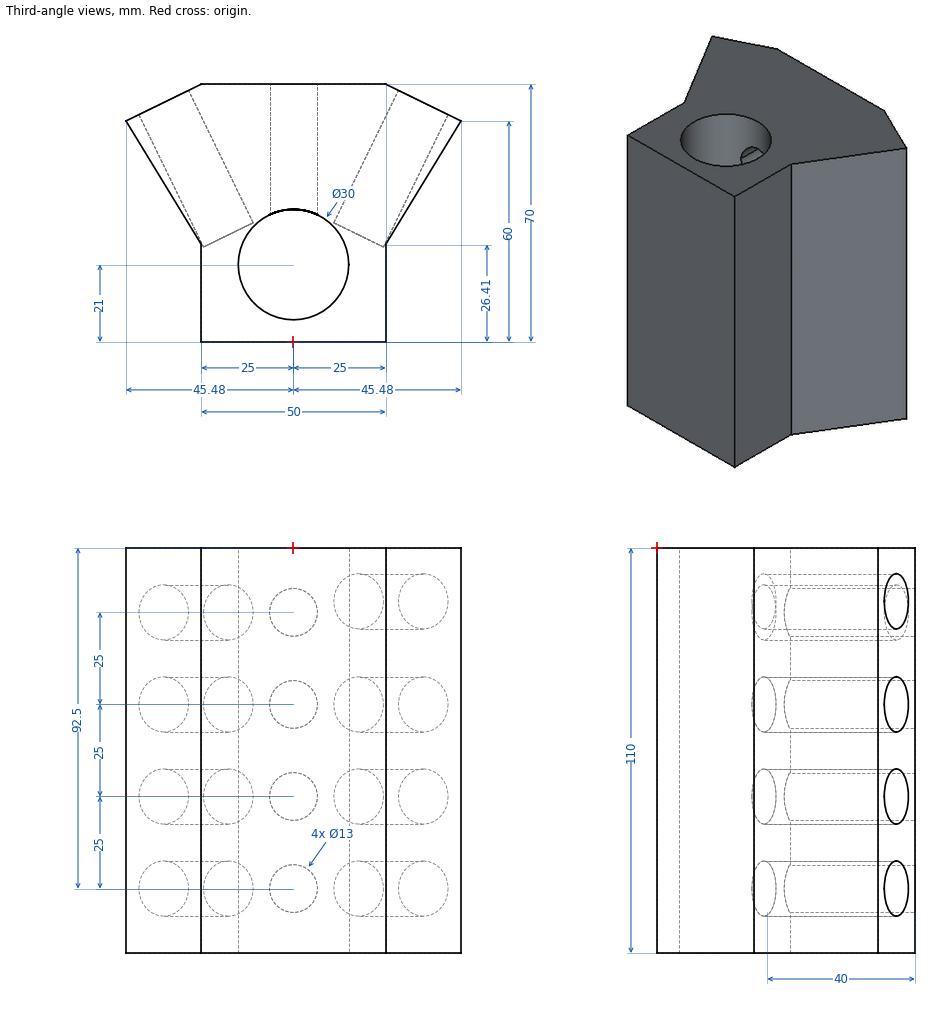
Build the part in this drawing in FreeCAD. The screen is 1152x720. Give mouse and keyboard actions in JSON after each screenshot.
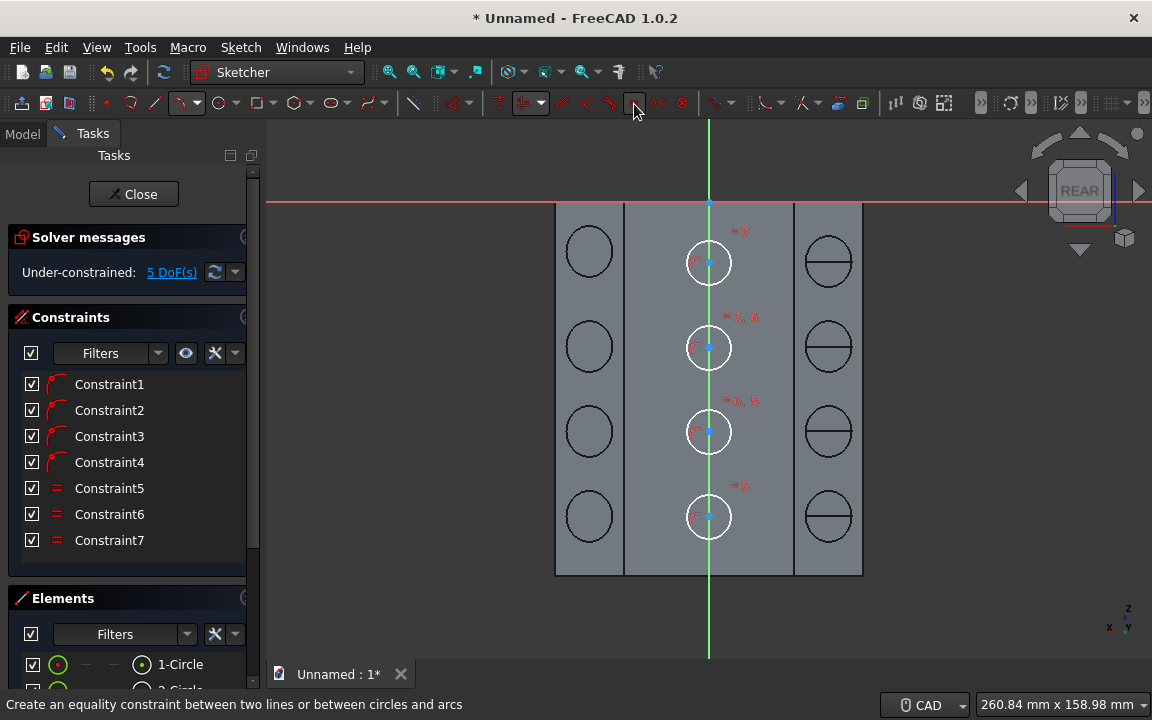
{"action": "left_click", "coordinate": [452, 104]}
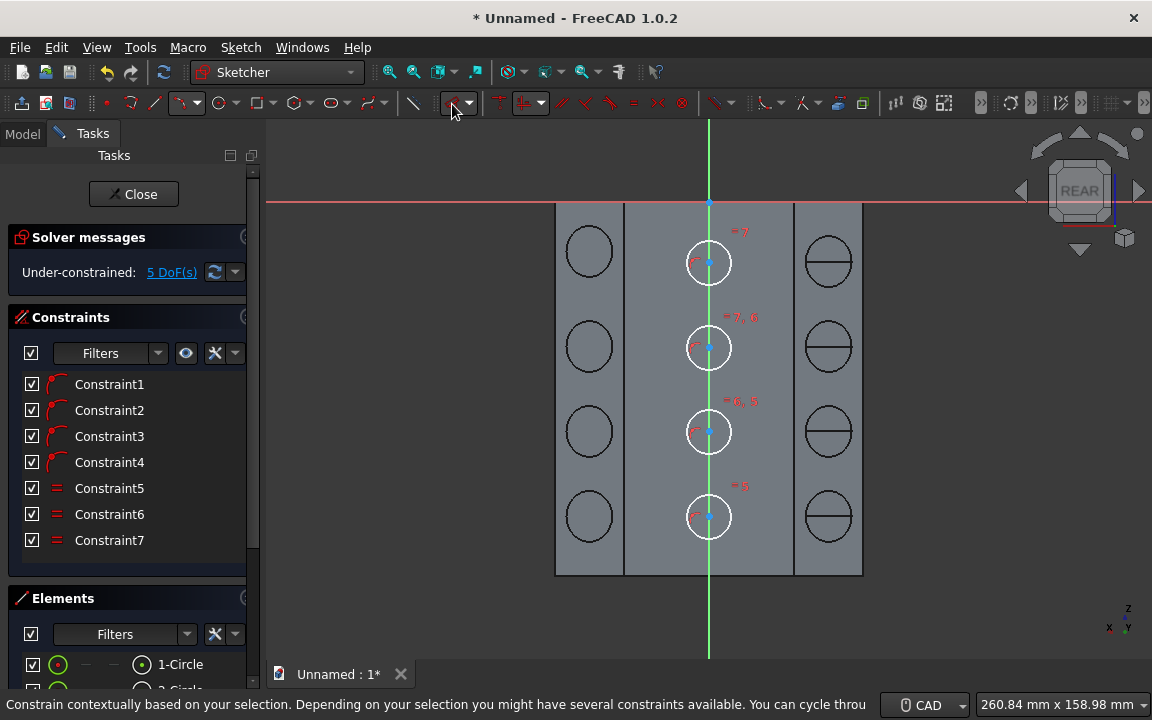
{"action": "left_click", "coordinate": [724, 501]}
{"action": "left_click", "coordinate": [746, 478]}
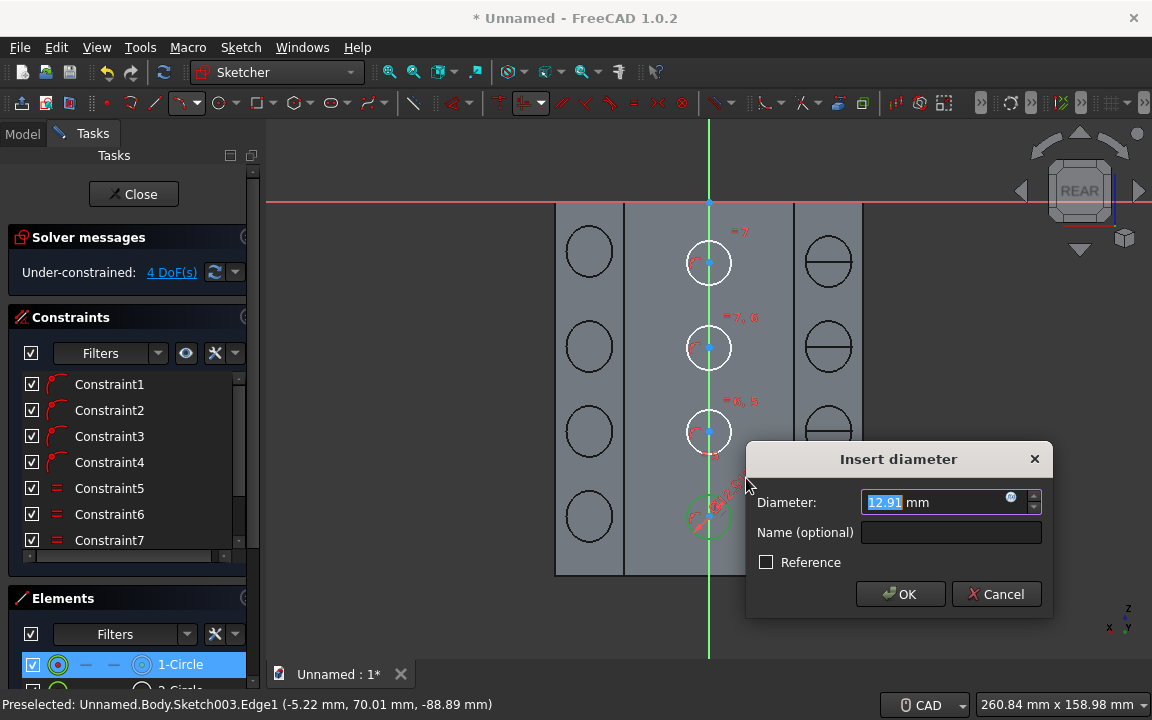
{"action": "type", "text": "13"}
{"action": "key", "text": "Return"}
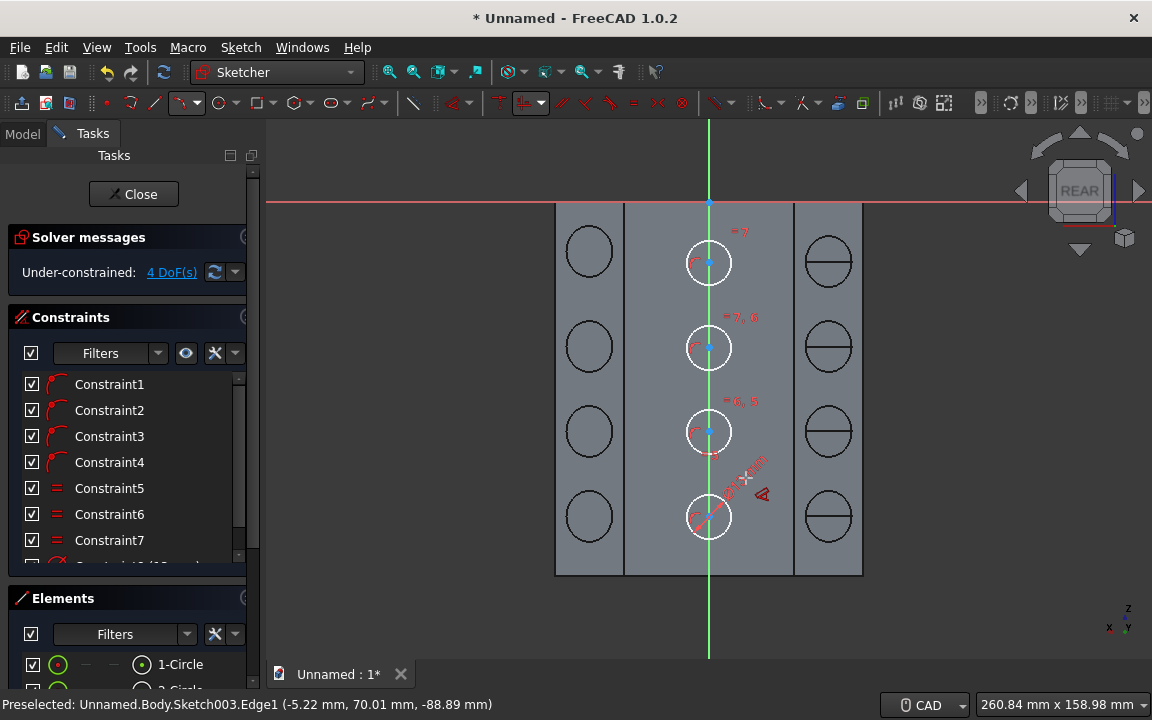
{"action": "left_click", "coordinate": [709, 517]}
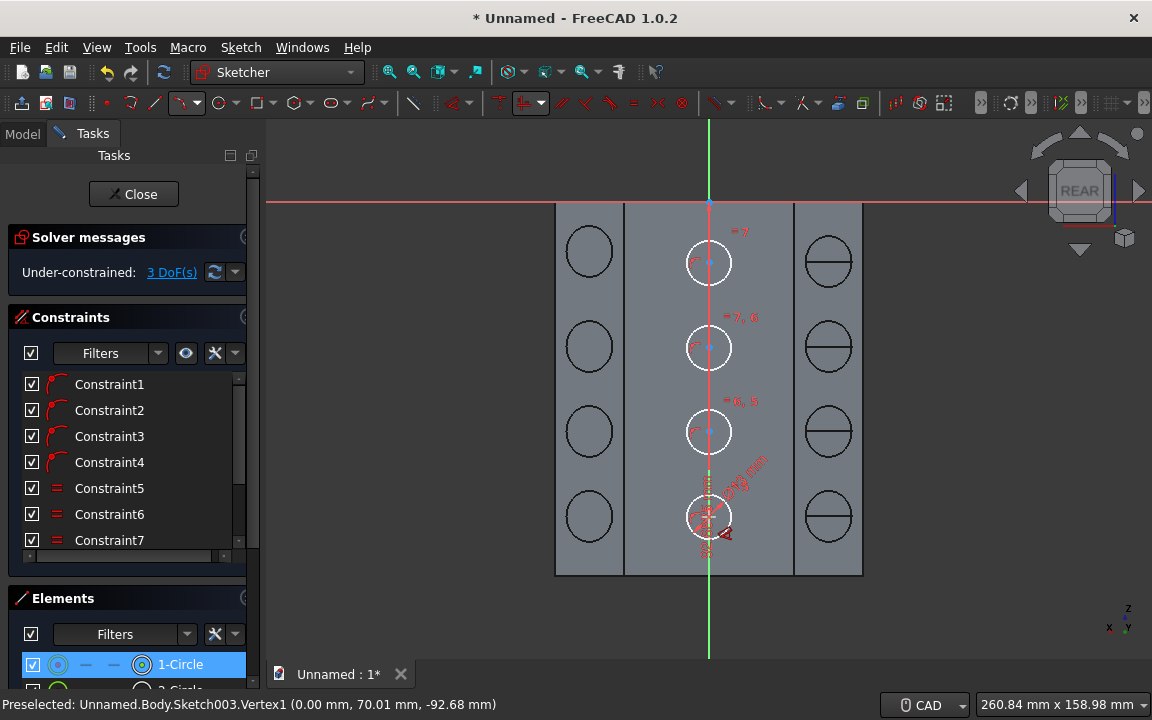
{"action": "left_click", "coordinate": [709, 432]}
{"action": "left_click", "coordinate": [743, 455]}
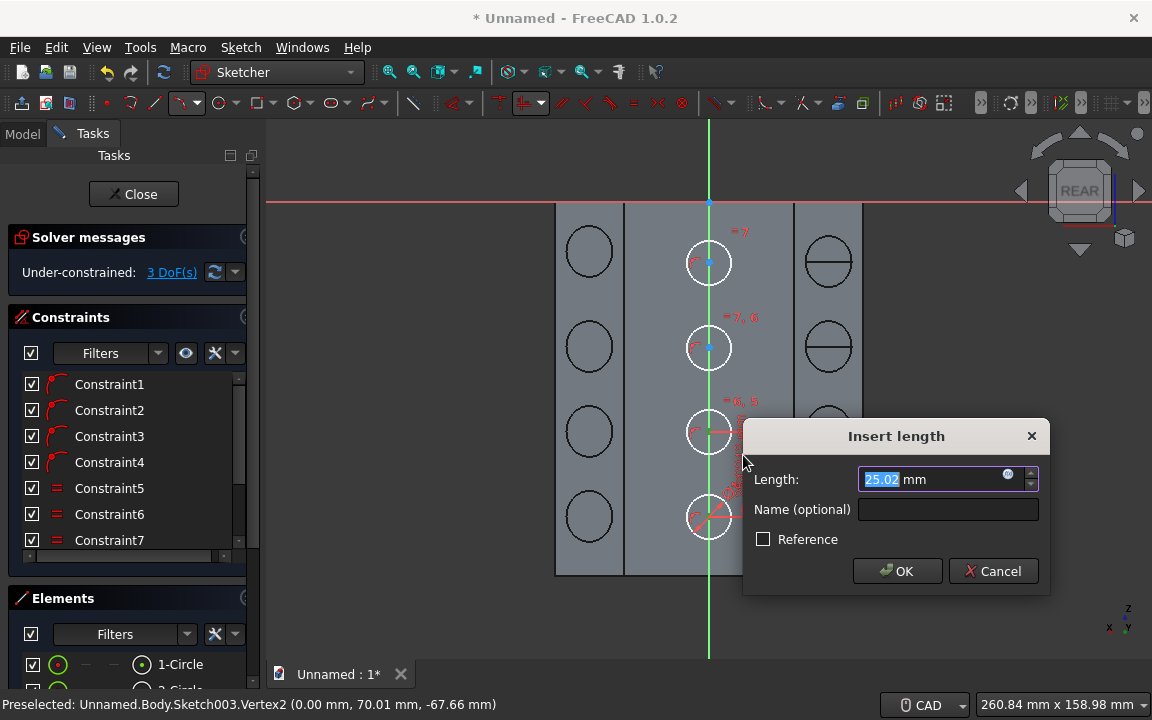
{"action": "type", "text": "25"}
{"action": "key", "text": "Return"}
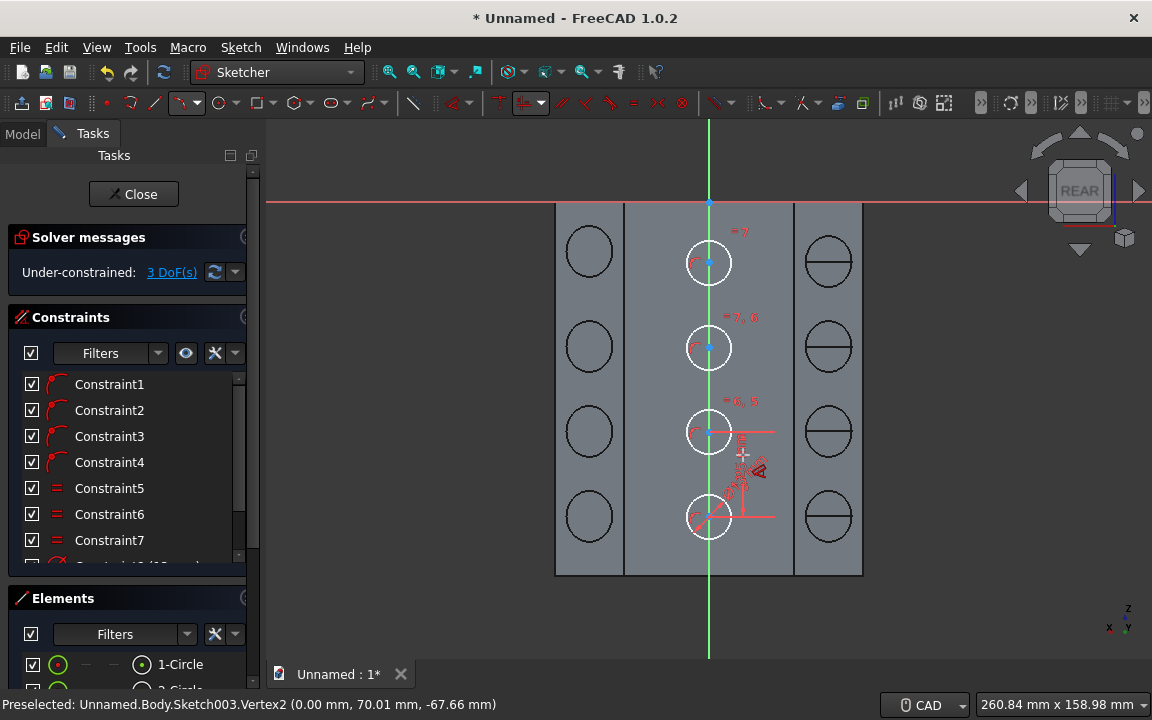
{"action": "left_click", "coordinate": [709, 432]}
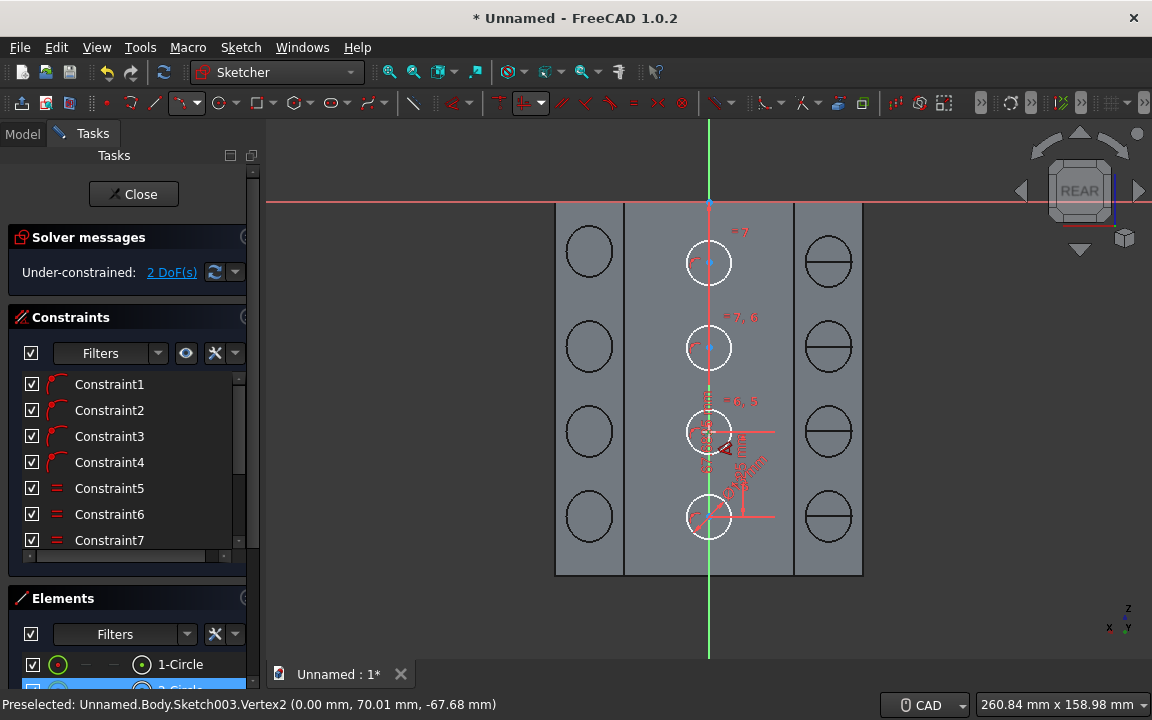
{"action": "left_click", "coordinate": [709, 348]}
{"action": "left_click", "coordinate": [743, 390]}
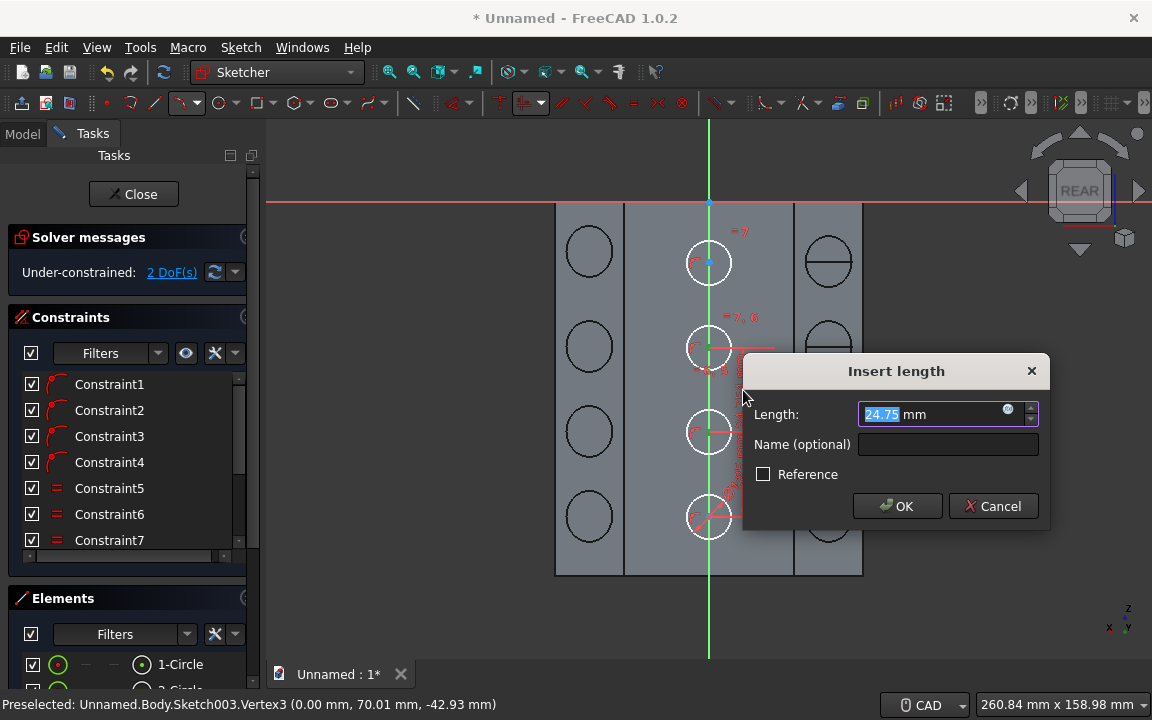
{"action": "type", "text": "25"}
{"action": "key", "text": "Return"}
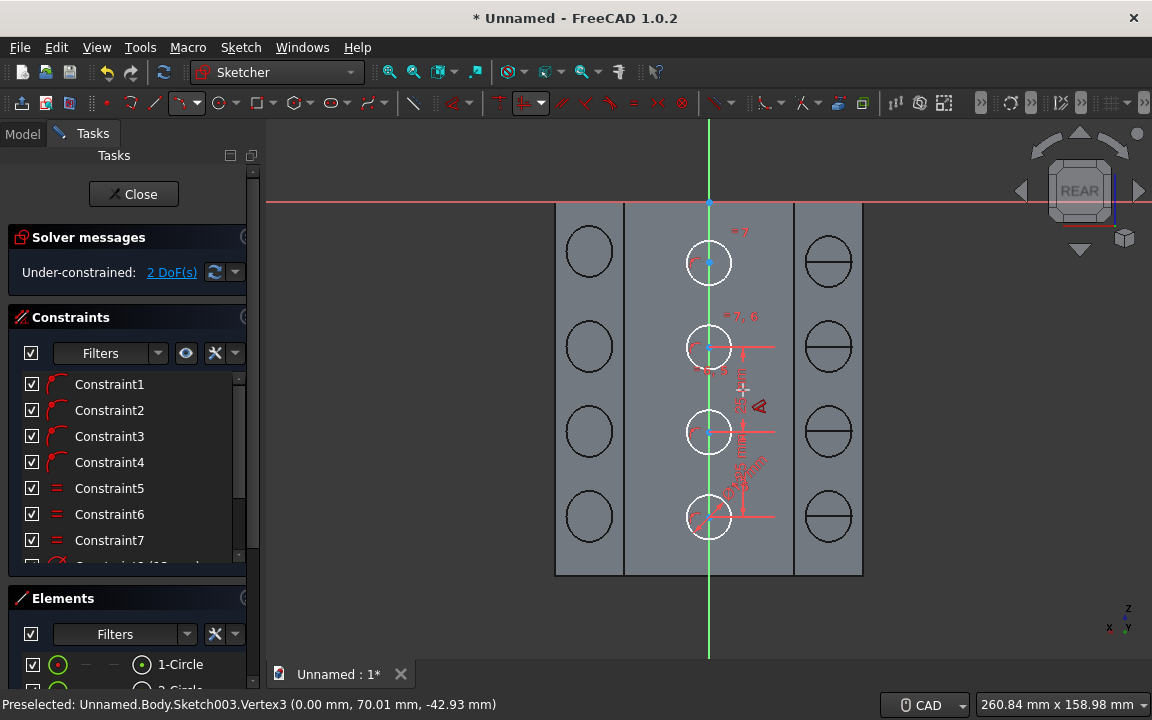
{"action": "left_click", "coordinate": [709, 347]}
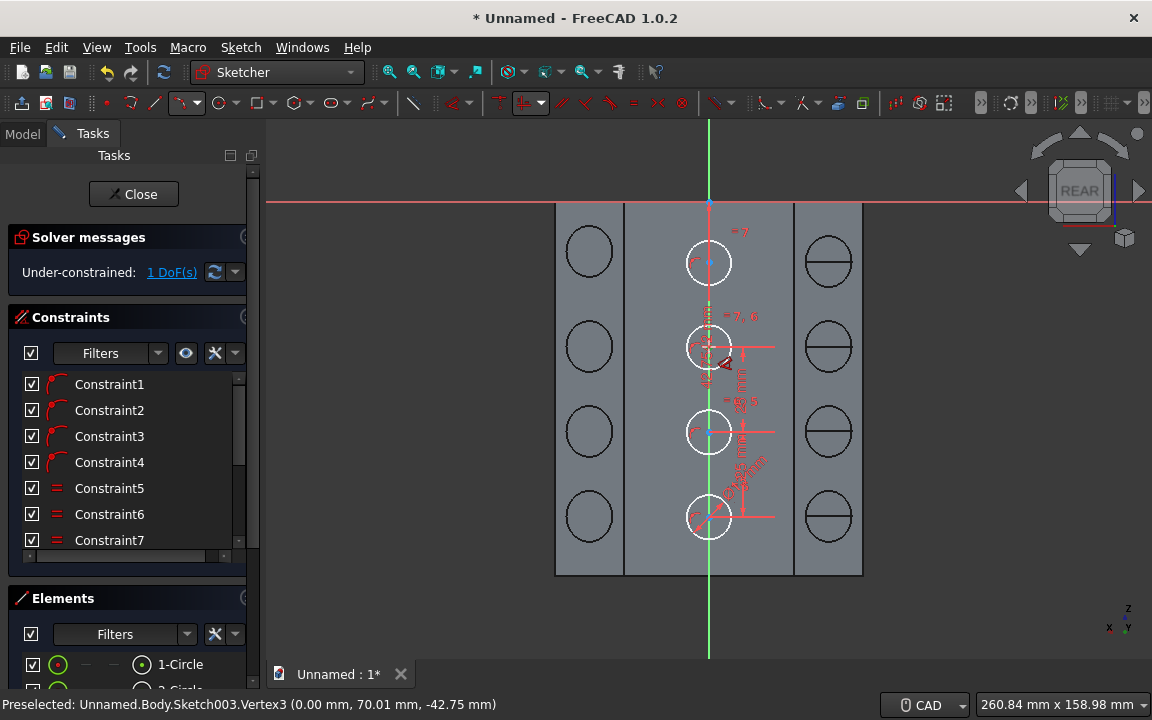
{"action": "left_click", "coordinate": [709, 263]}
{"action": "left_click", "coordinate": [743, 305]}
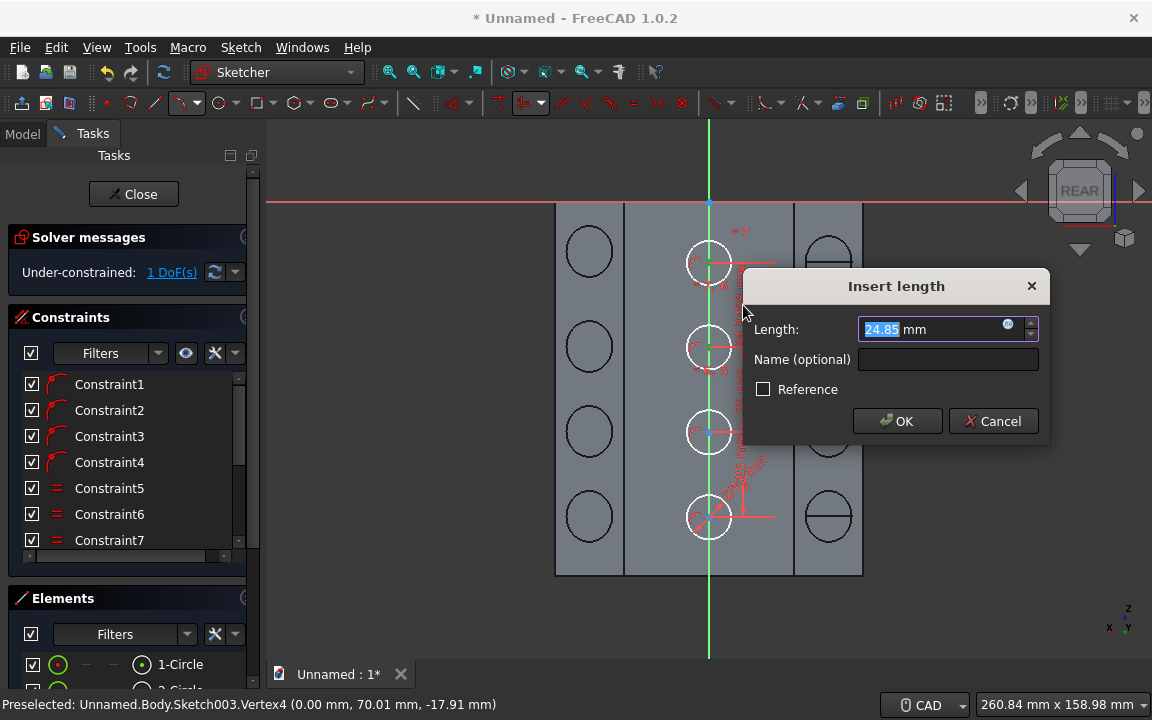
{"action": "type", "text": "25"}
{"action": "key", "text": "Return"}